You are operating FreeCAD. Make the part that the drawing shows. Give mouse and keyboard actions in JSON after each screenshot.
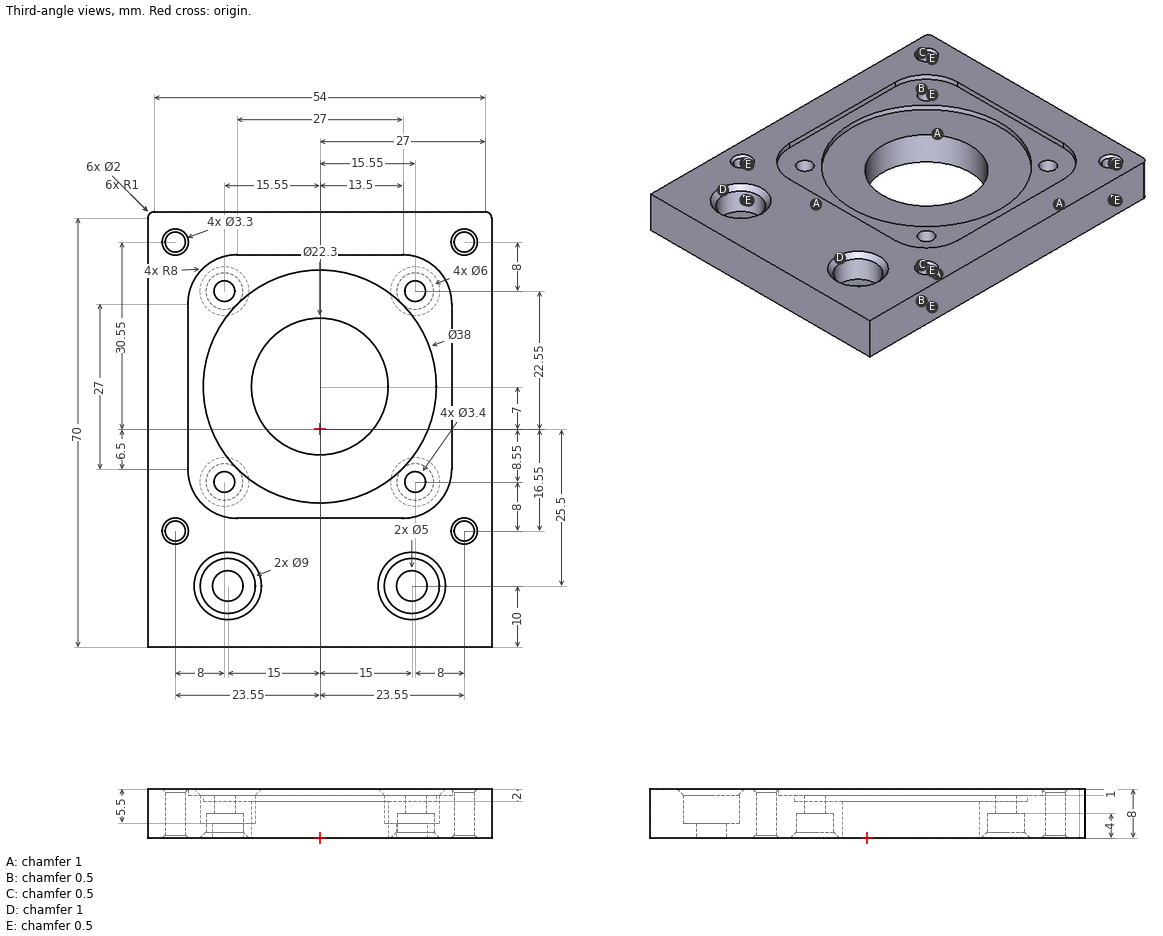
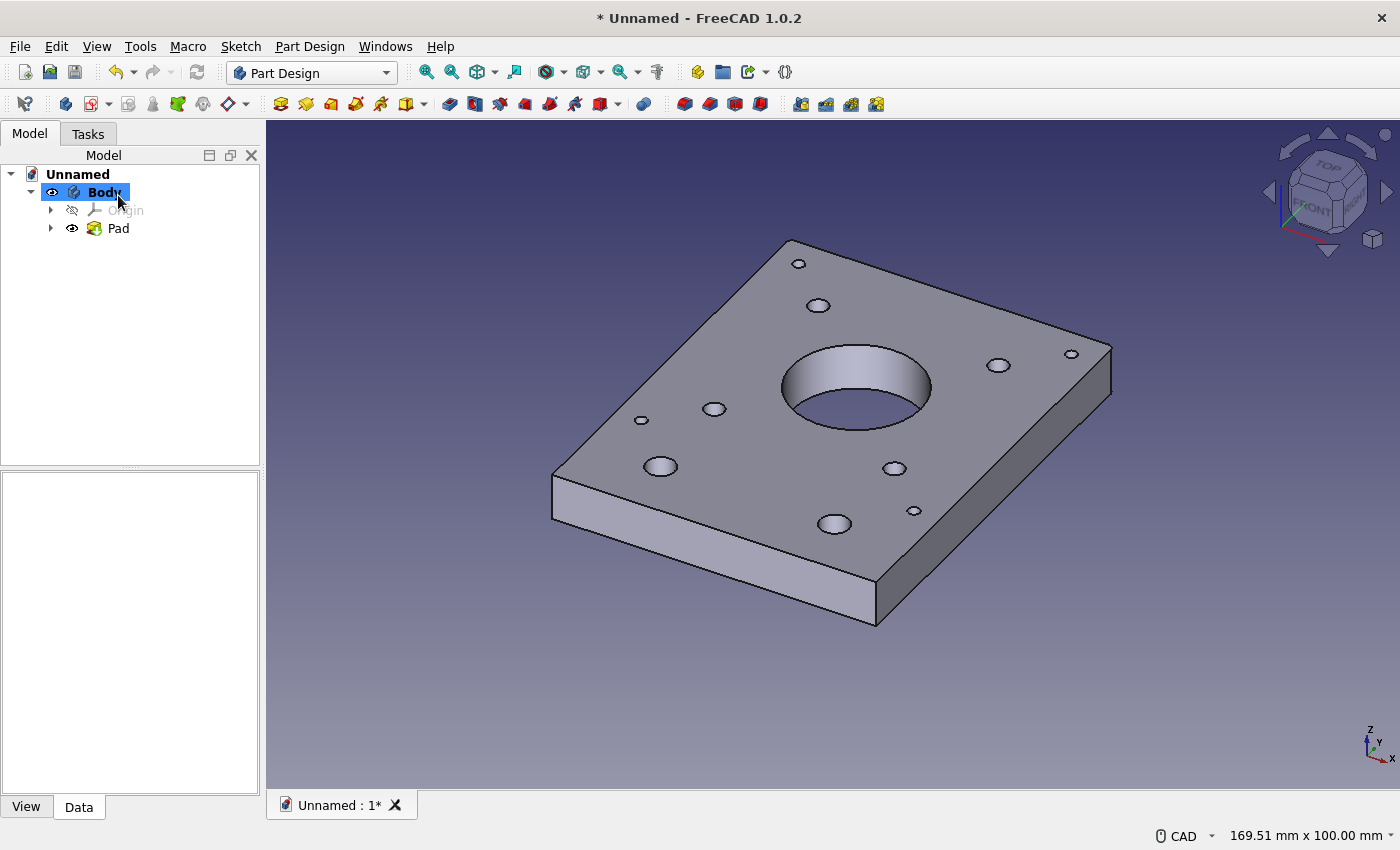
{"action": "left_click", "coordinate": [765, 477]}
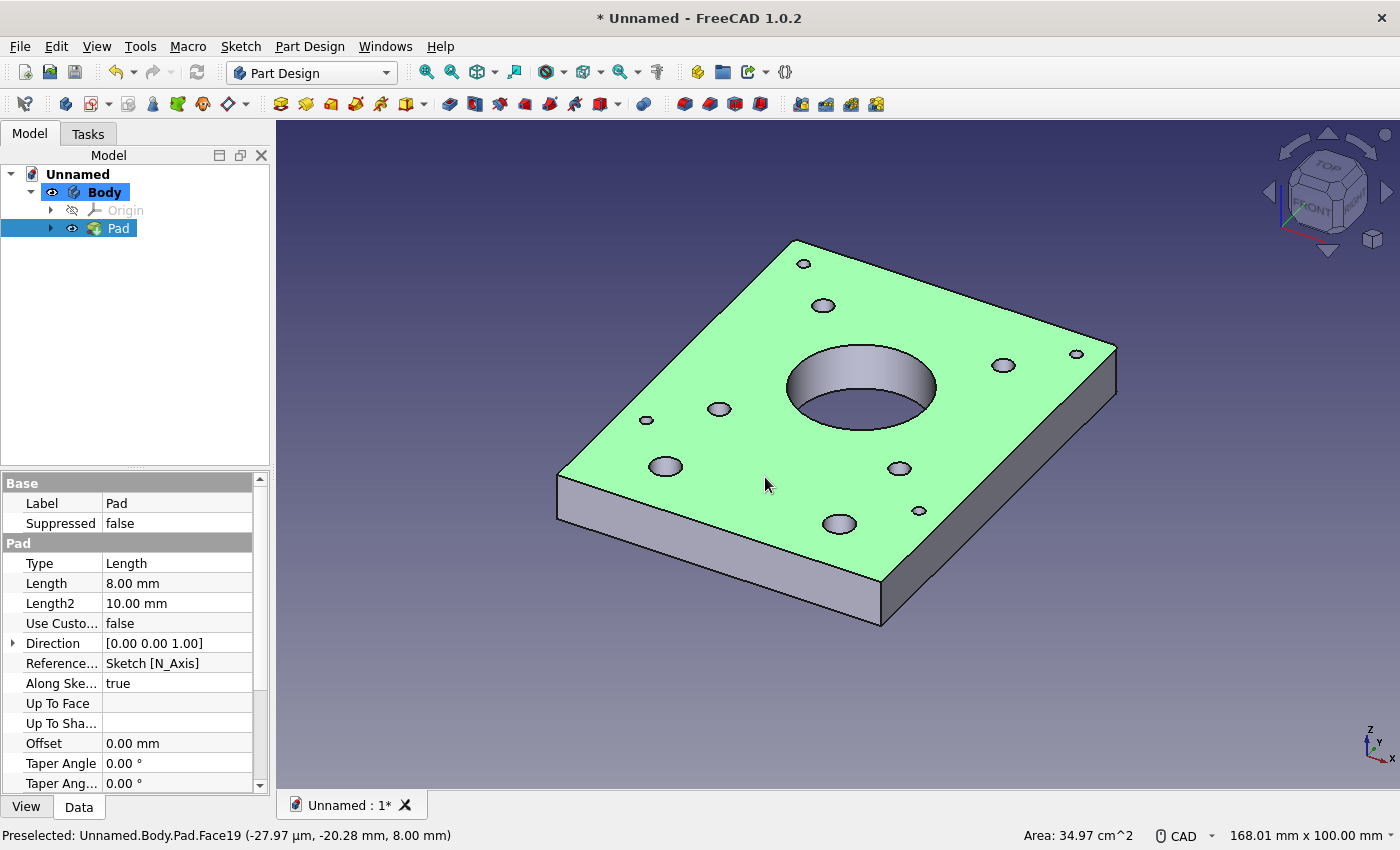
{"action": "left_click", "coordinate": [90, 104]}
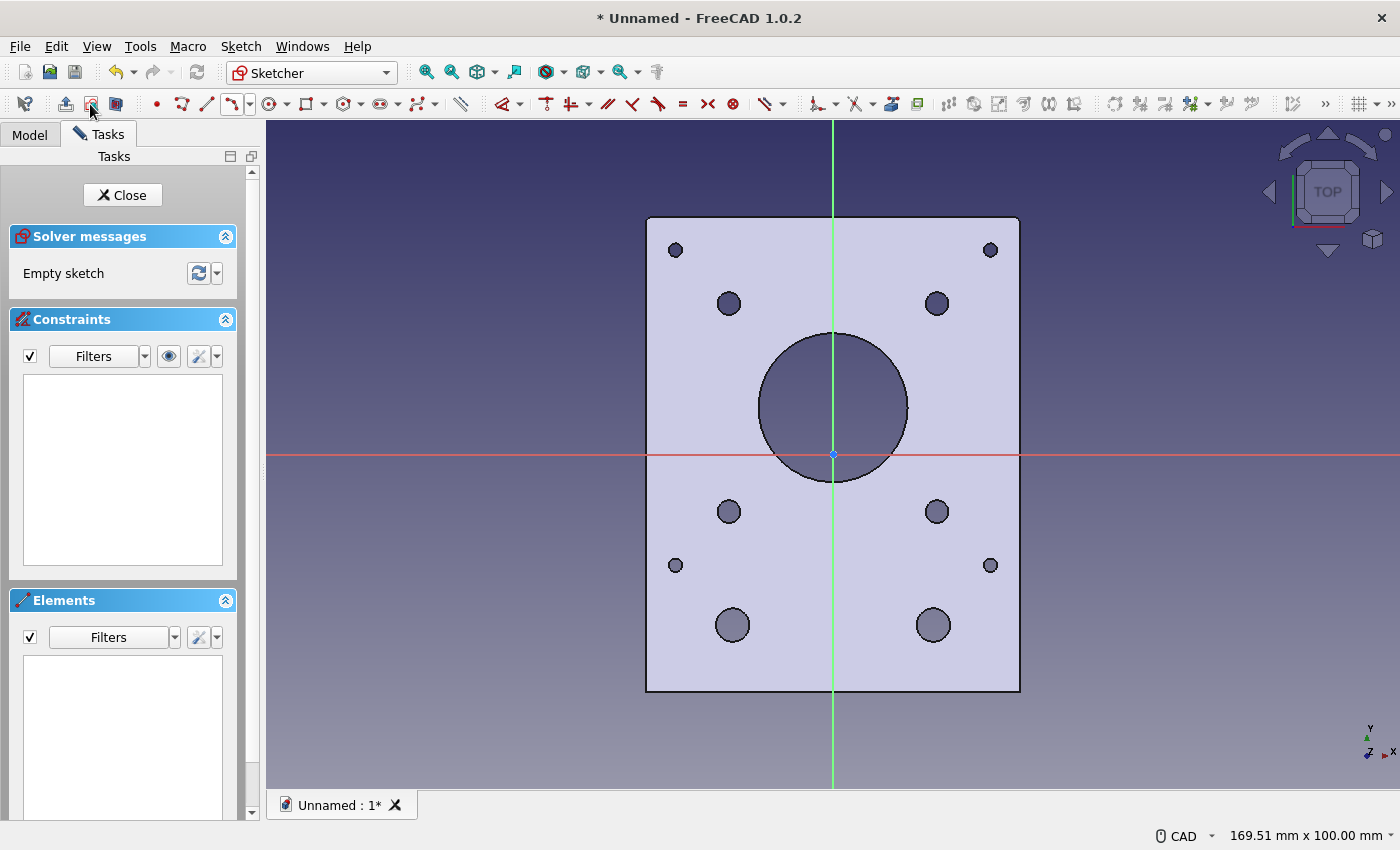
{"action": "scroll", "coordinate": [889, 637], "scroll_direction": "up", "scroll_amount": 4}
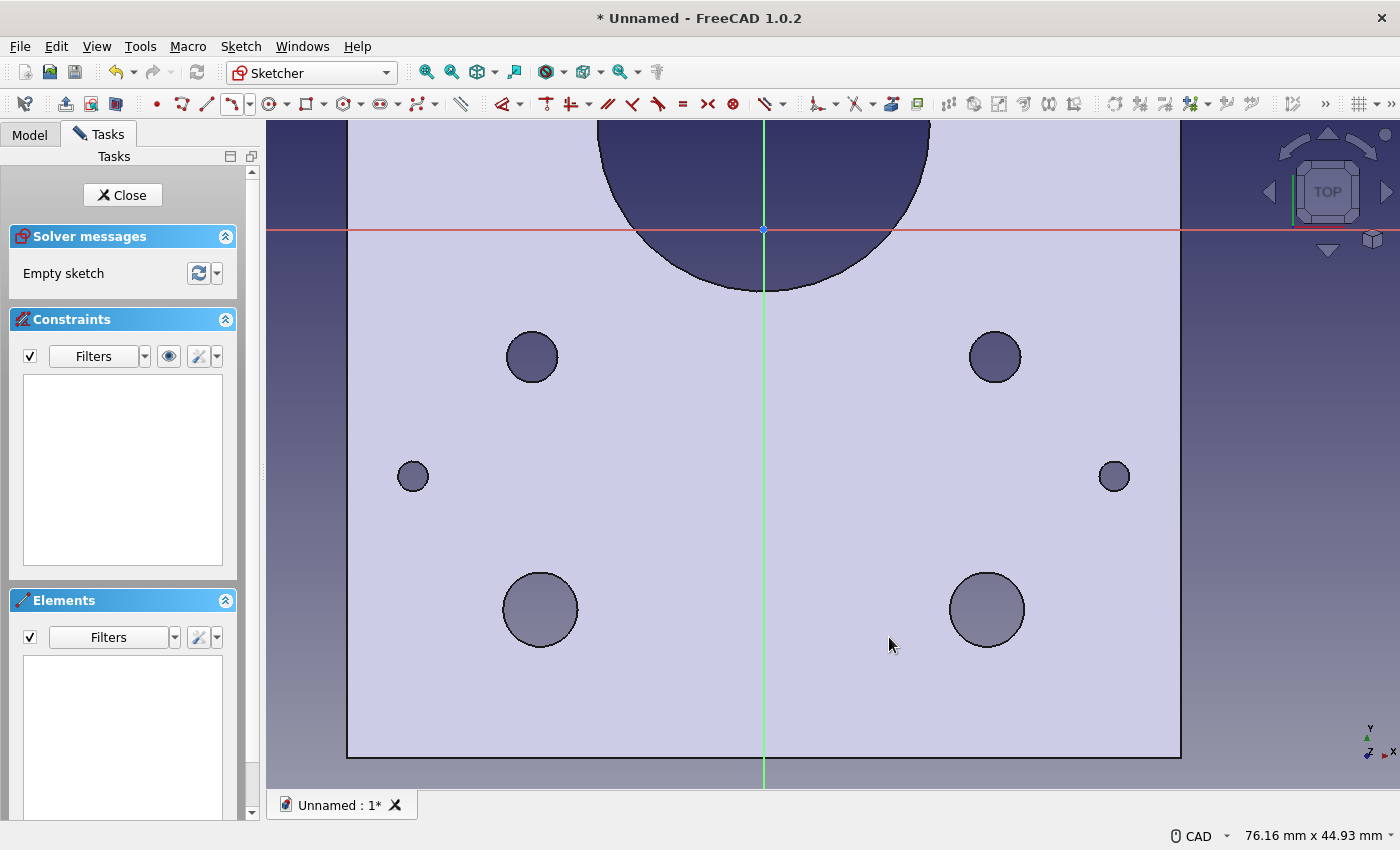
{"action": "key", "text": "g c"}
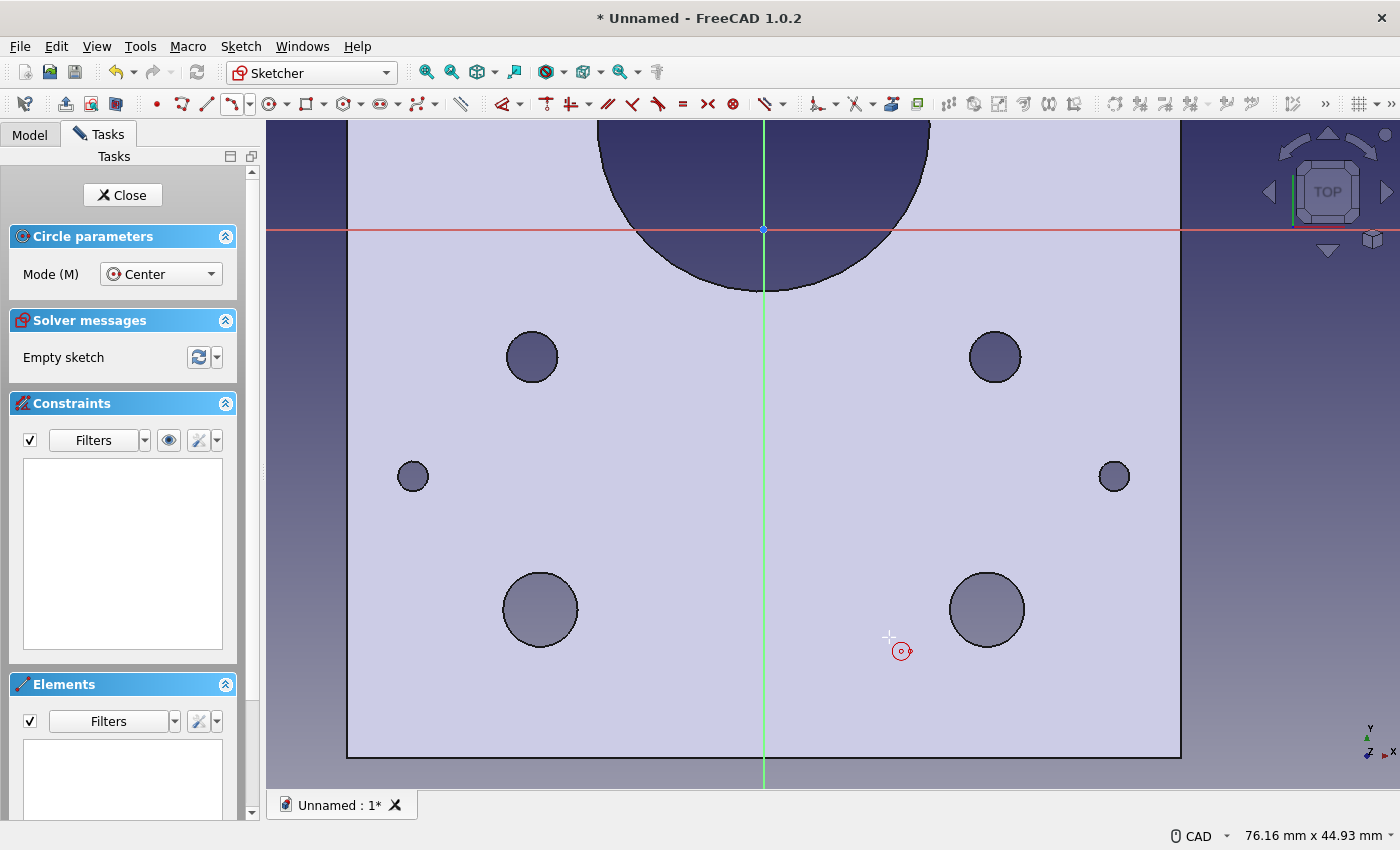
{"action": "left_click", "coordinate": [540, 610]}
{"action": "left_click", "coordinate": [588, 562]}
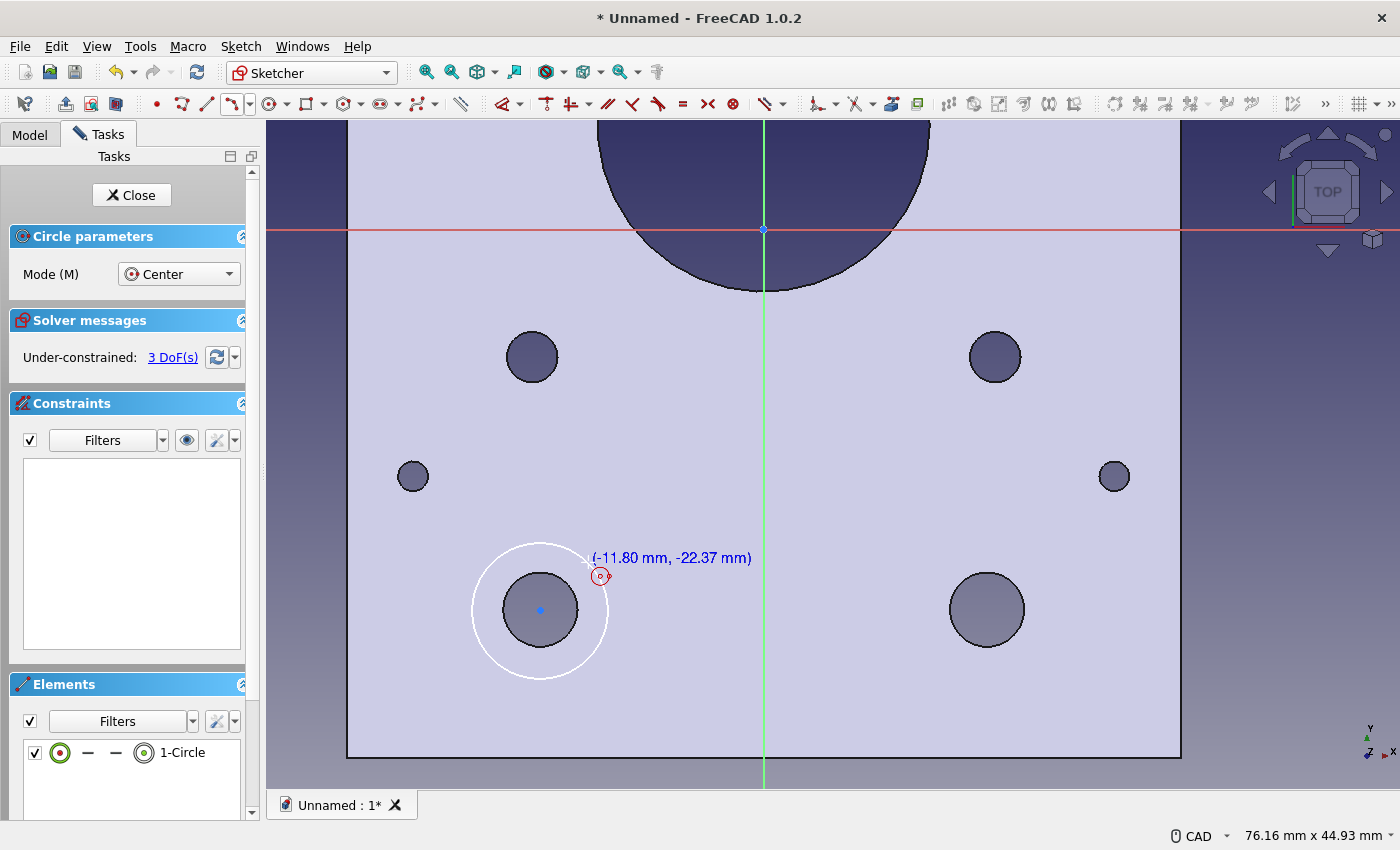
{"action": "left_click", "coordinate": [987, 610]}
{"action": "left_click", "coordinate": [1034, 562]}
{"action": "key", "text": "Escape"}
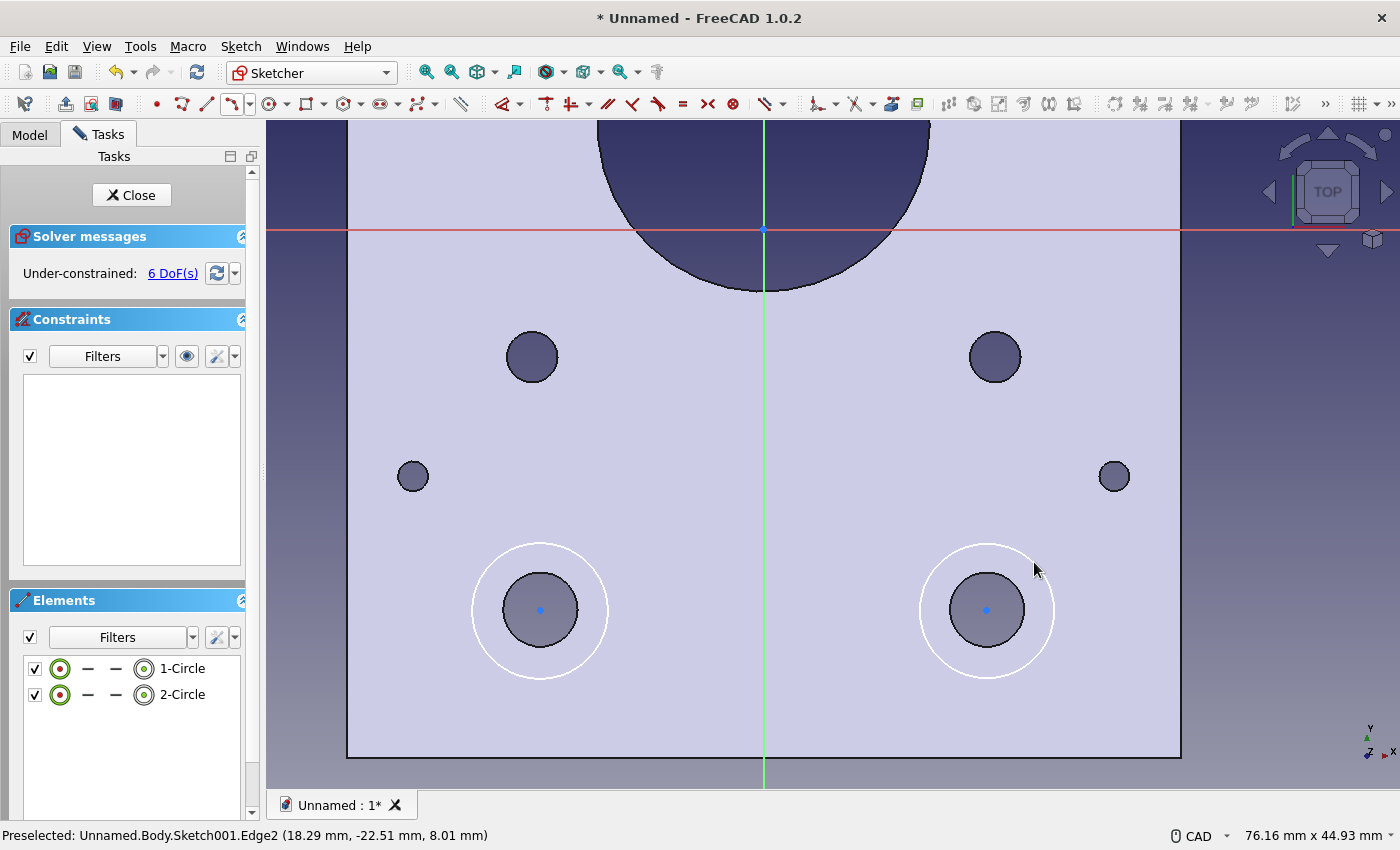
{"action": "left_click", "coordinate": [588, 563]}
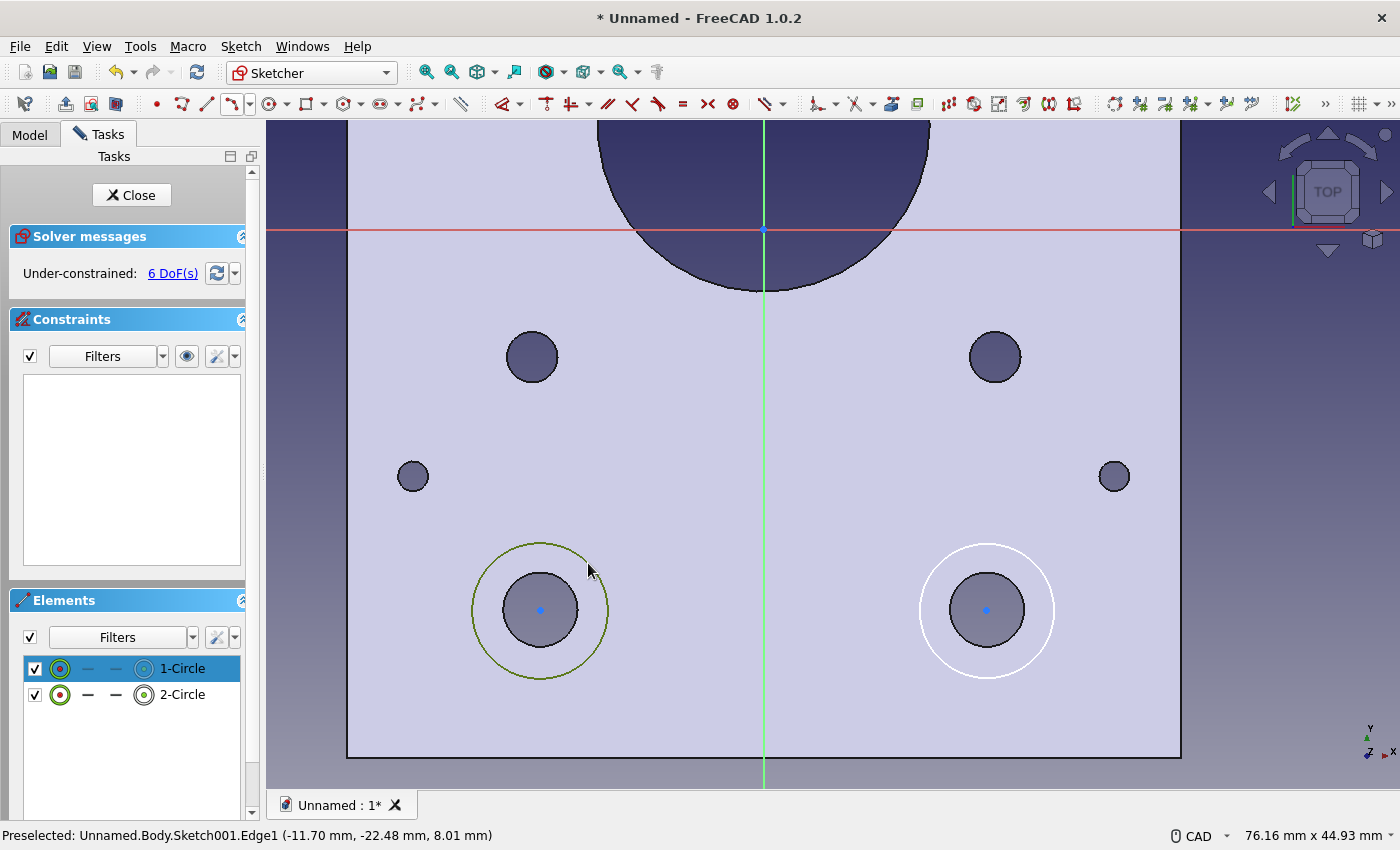
{"action": "left_click", "coordinate": [1034, 563]}